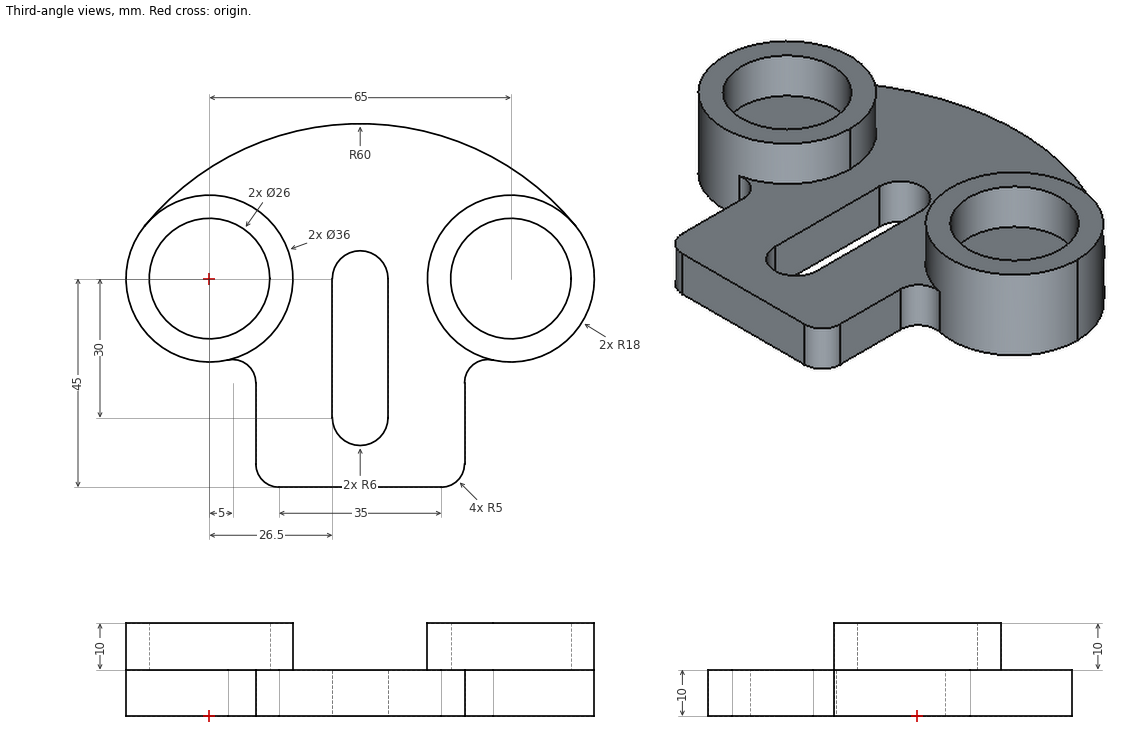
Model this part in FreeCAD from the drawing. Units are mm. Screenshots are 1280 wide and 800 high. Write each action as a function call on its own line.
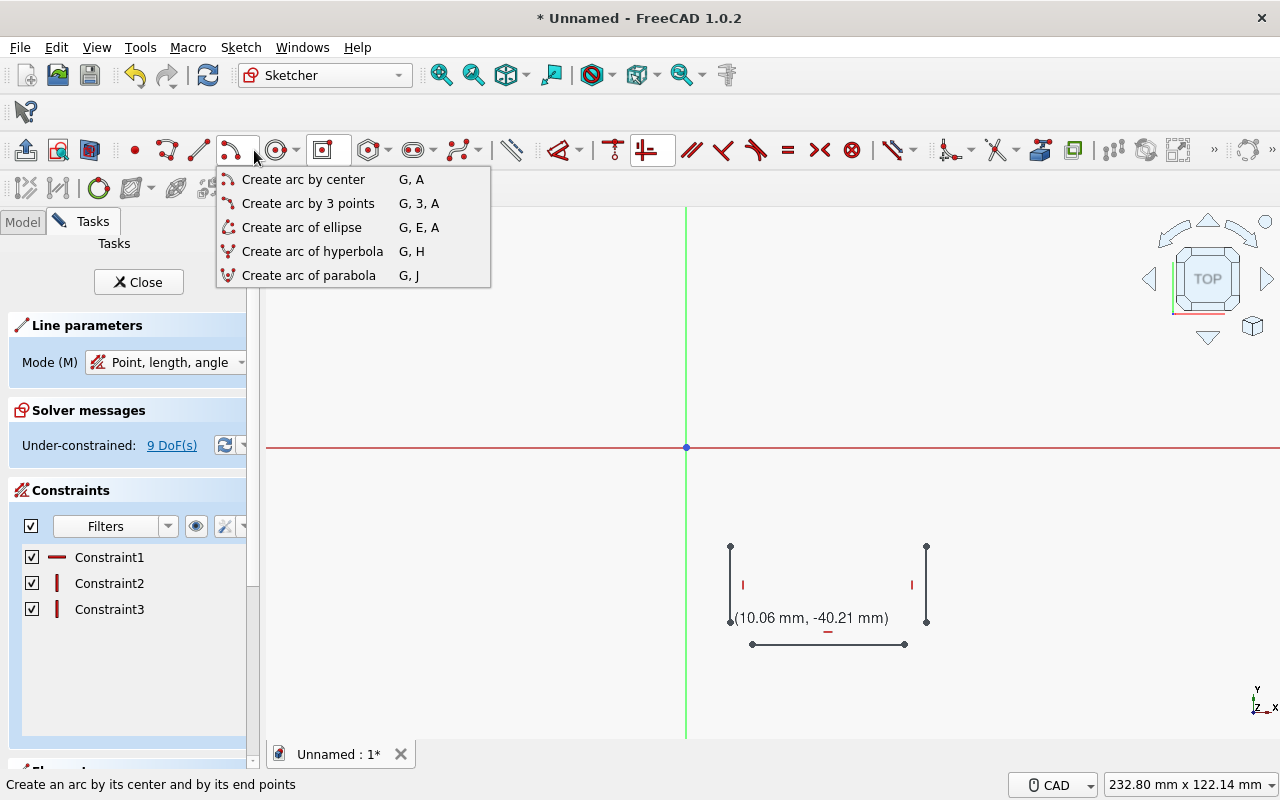
click(354, 203)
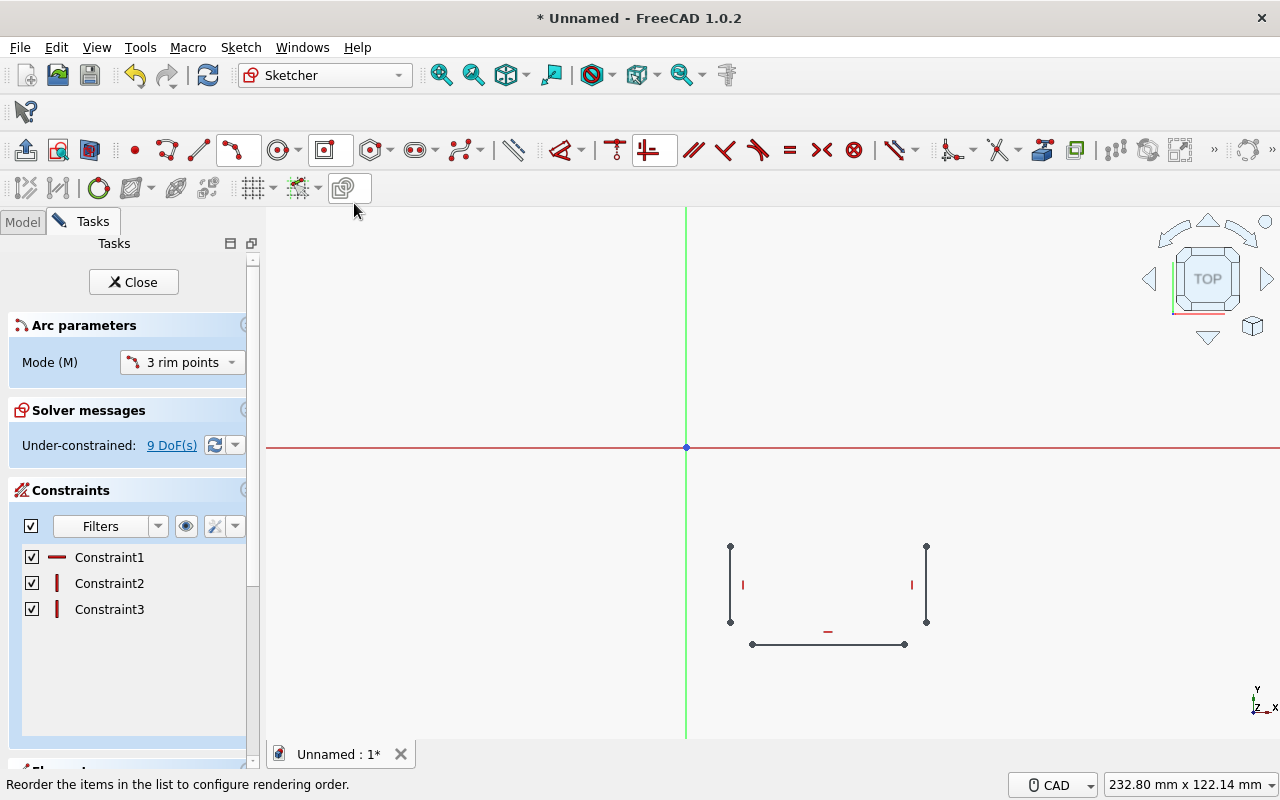
click(904, 645)
click(926, 623)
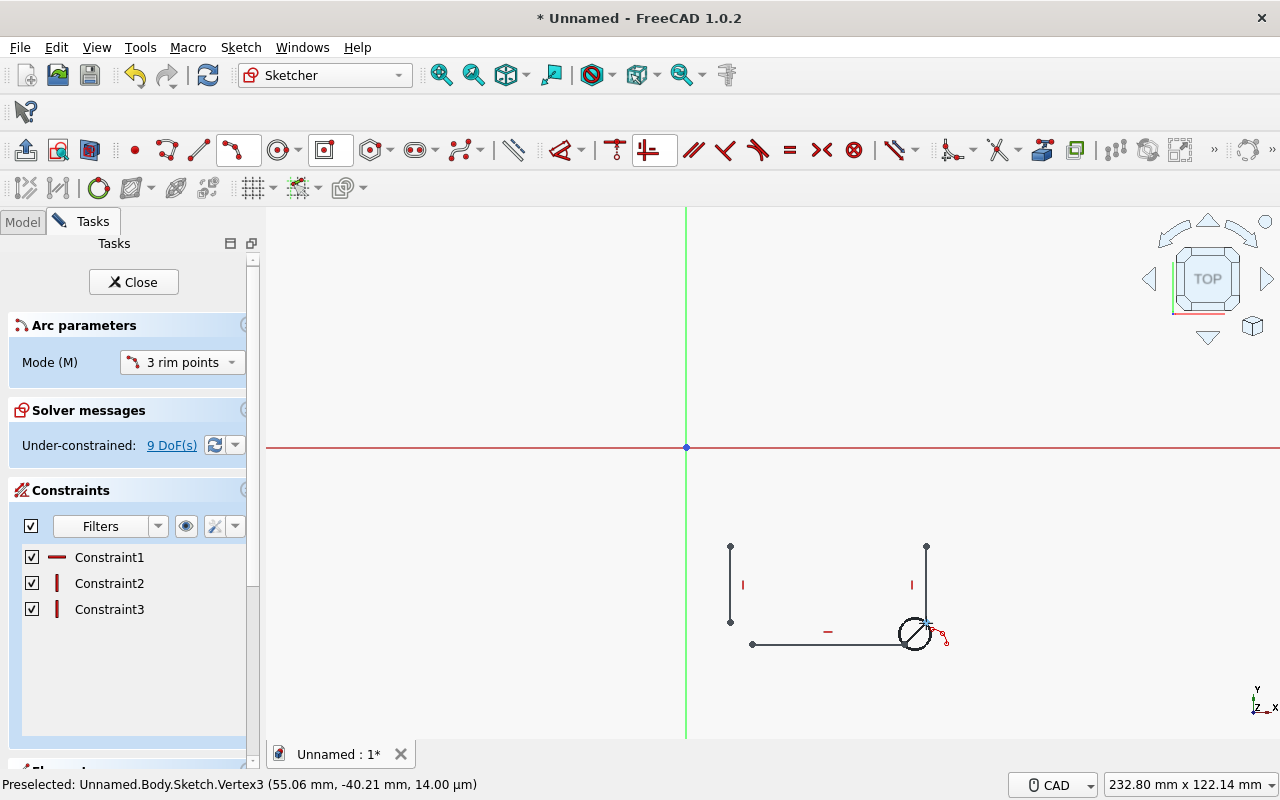
scroll(919, 637, up, 5)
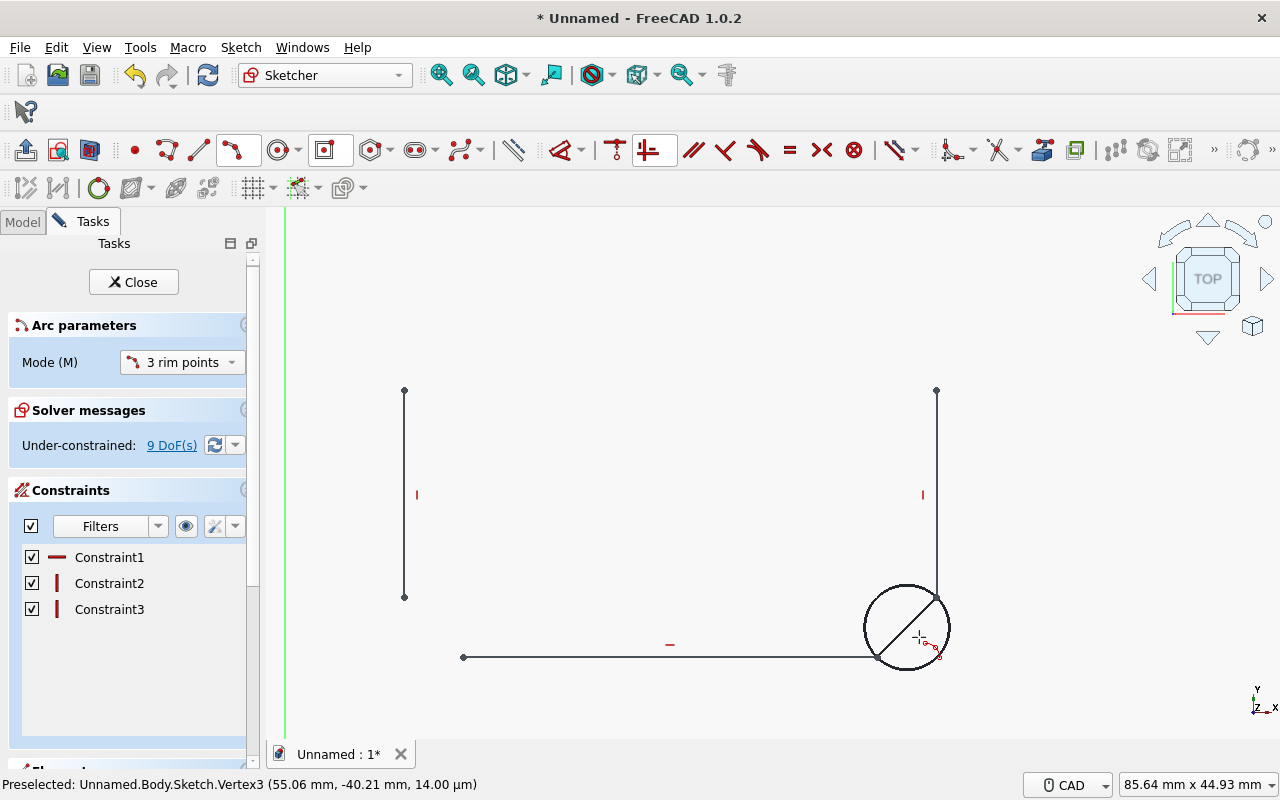
click(919, 637)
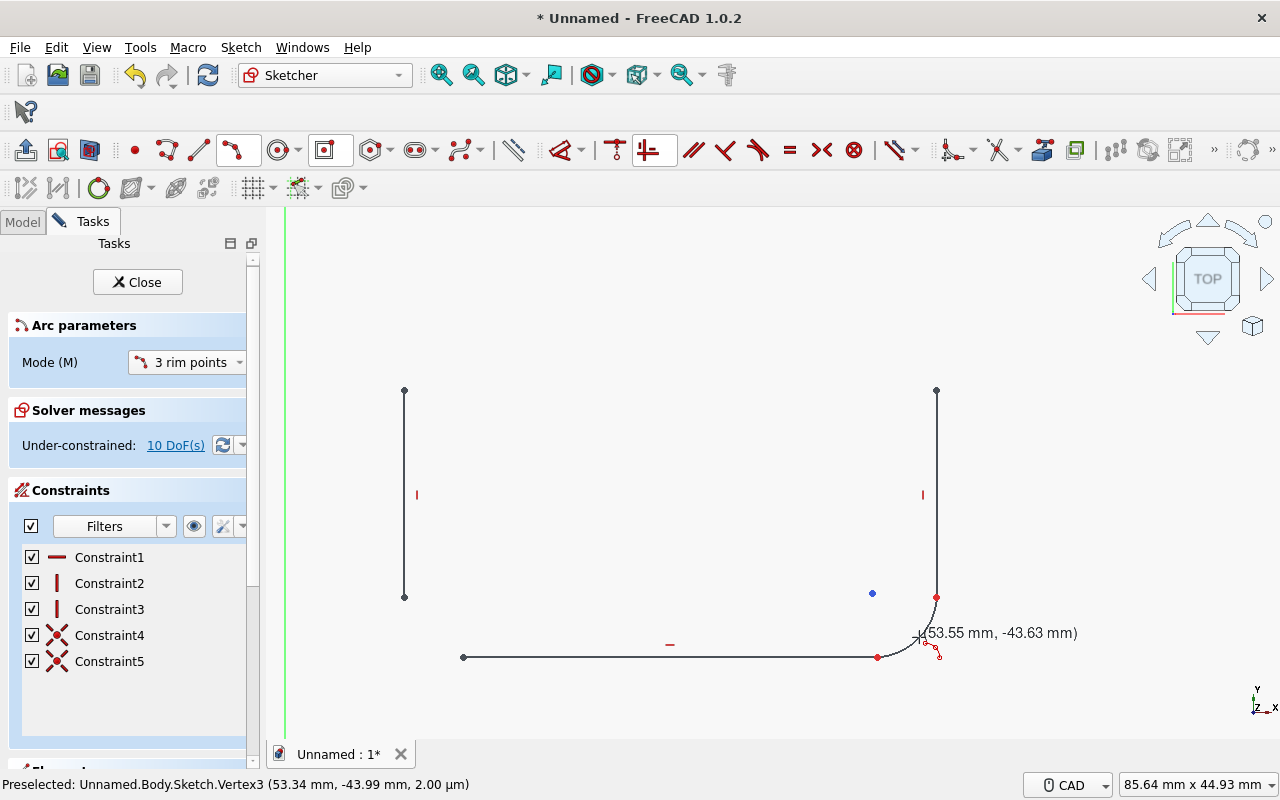
click(937, 391)
click(1008, 329)
click(958, 341)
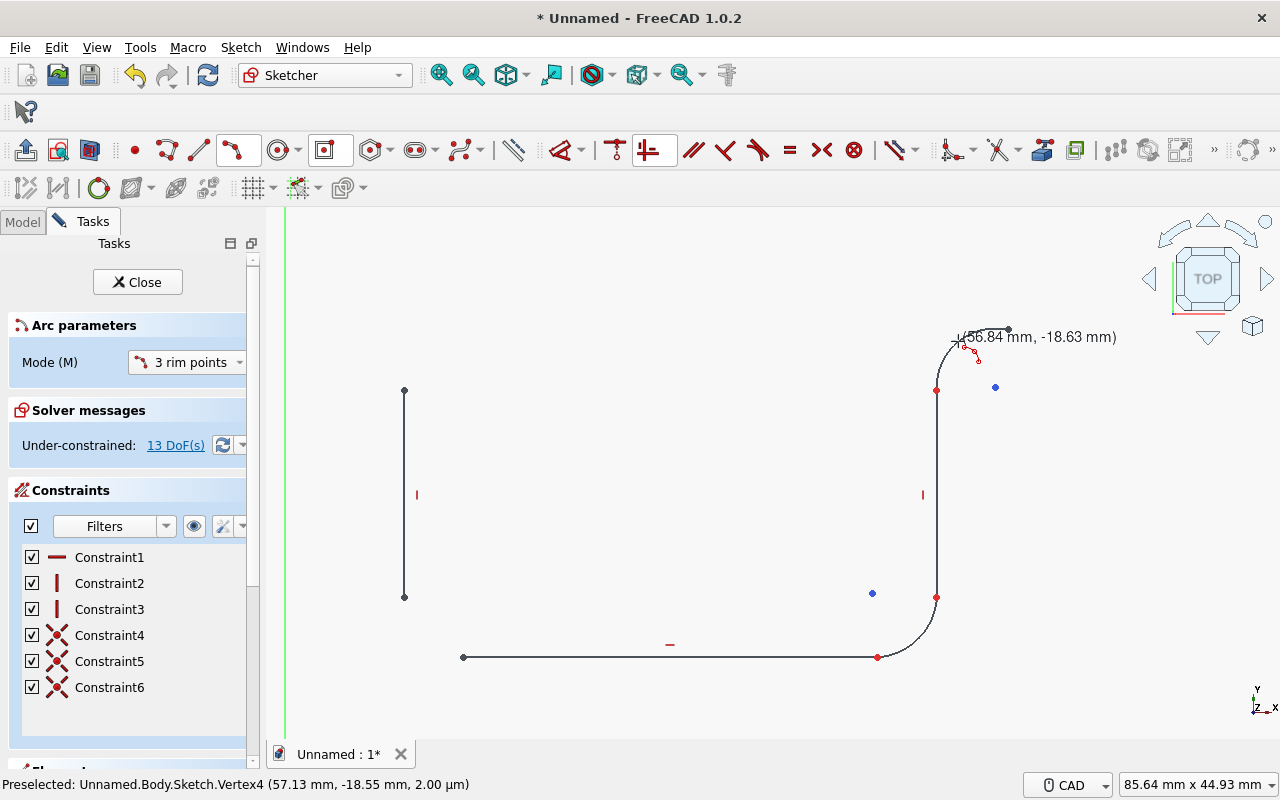
click(1008, 330)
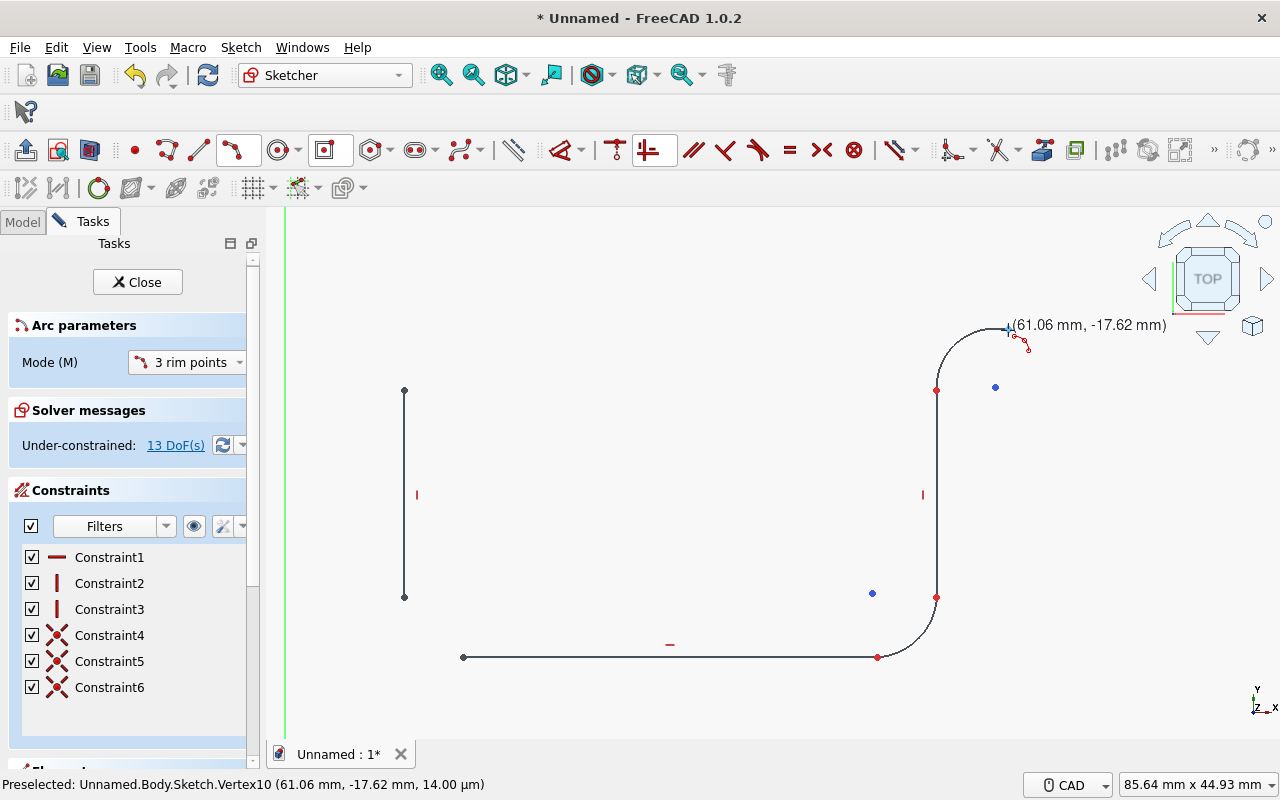
scroll(725, 638, down, 5)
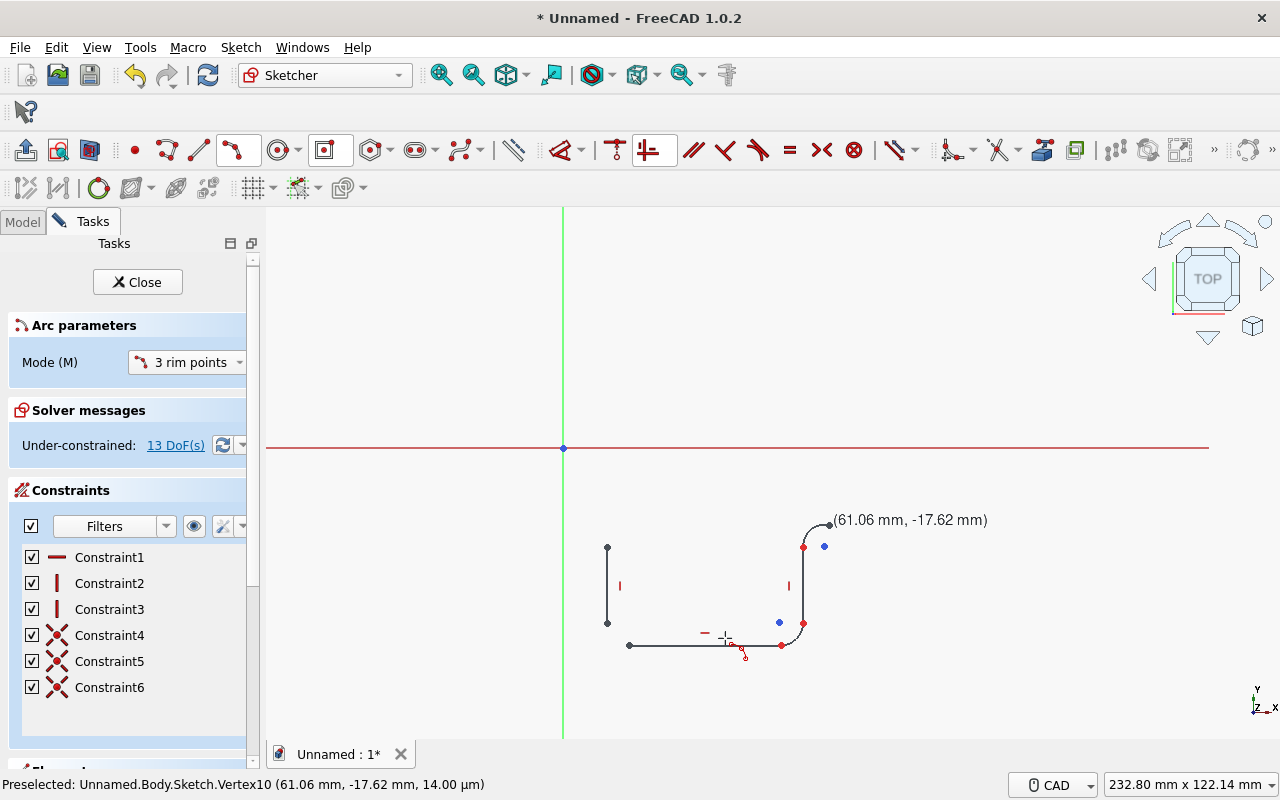
click(907, 399)
click(913, 490)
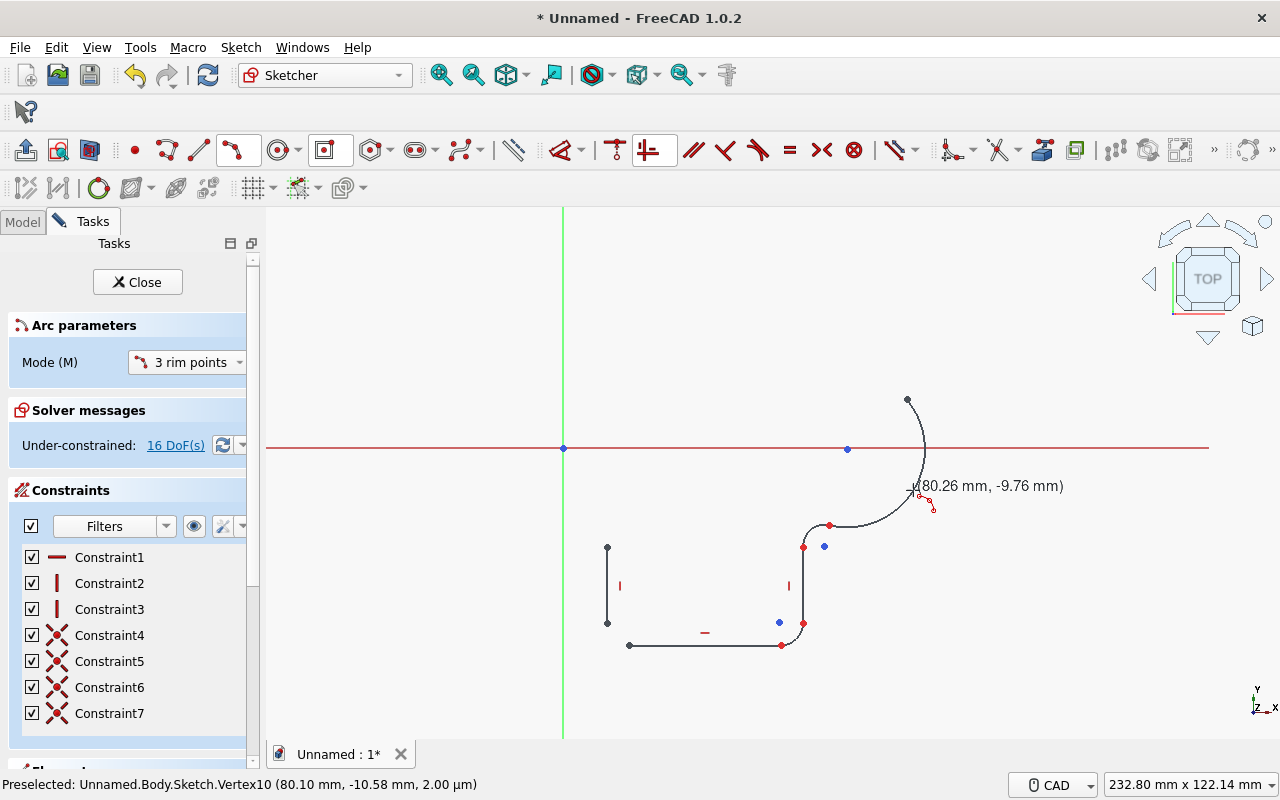
click(907, 400)
click(503, 399)
click(705, 303)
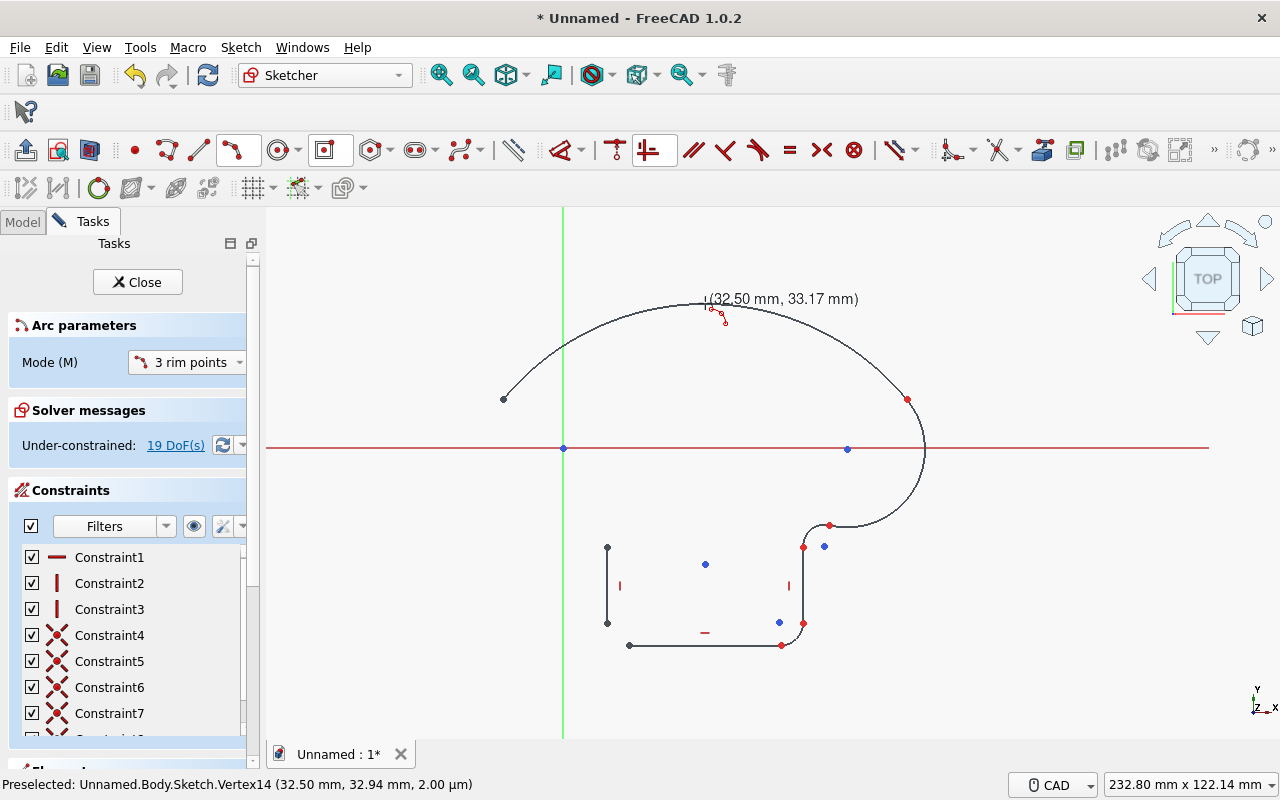
click(503, 400)
click(580, 525)
click(497, 490)